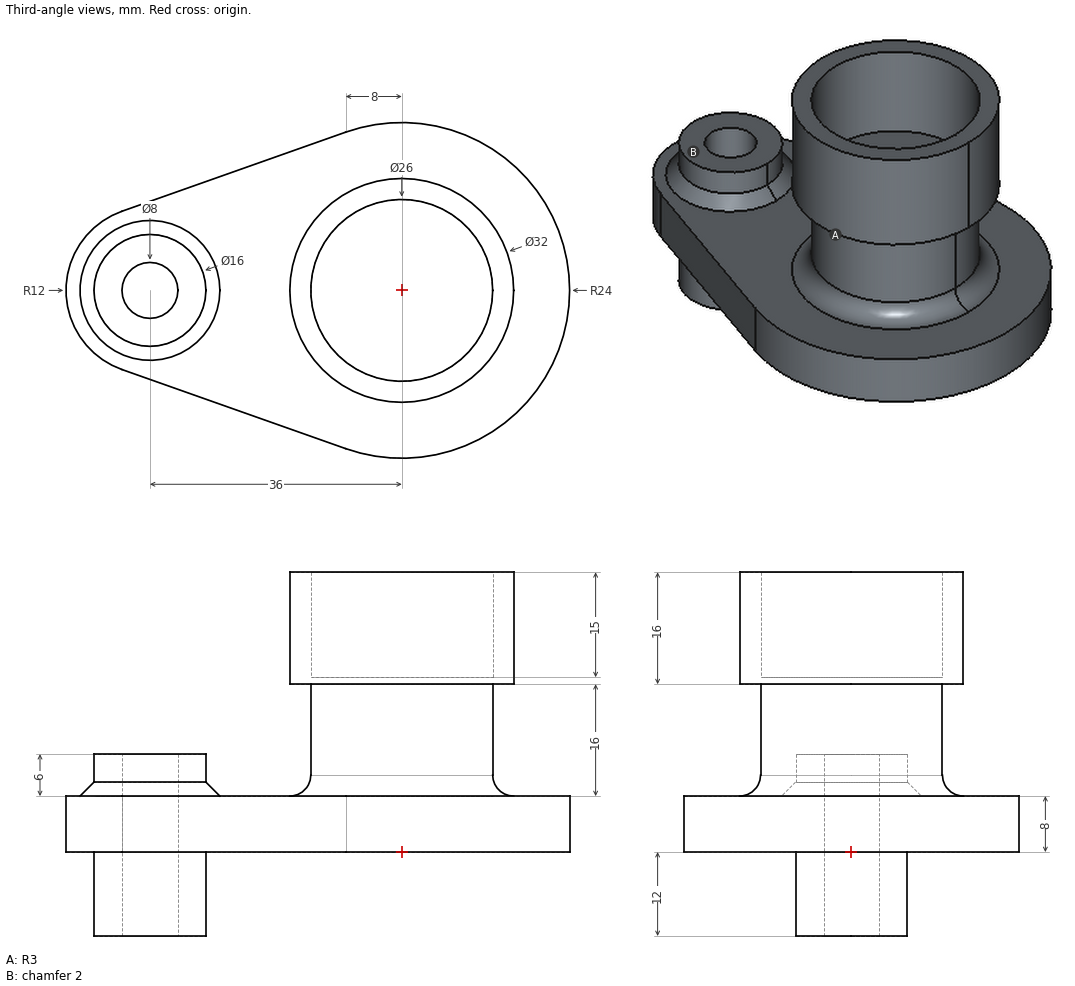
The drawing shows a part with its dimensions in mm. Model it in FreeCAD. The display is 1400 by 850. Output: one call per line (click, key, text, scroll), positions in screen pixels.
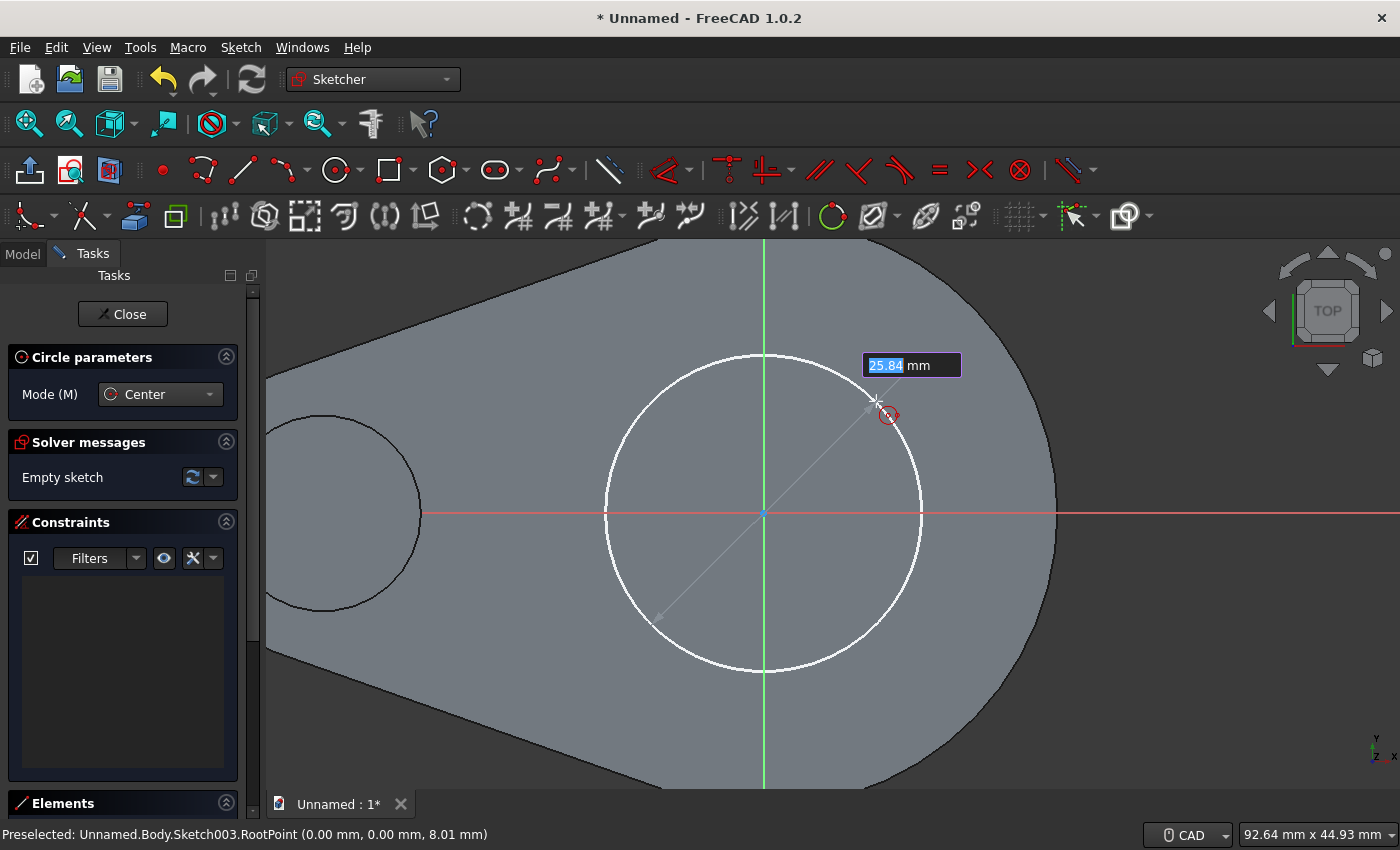
text(26)
key(Return)
key(Escape)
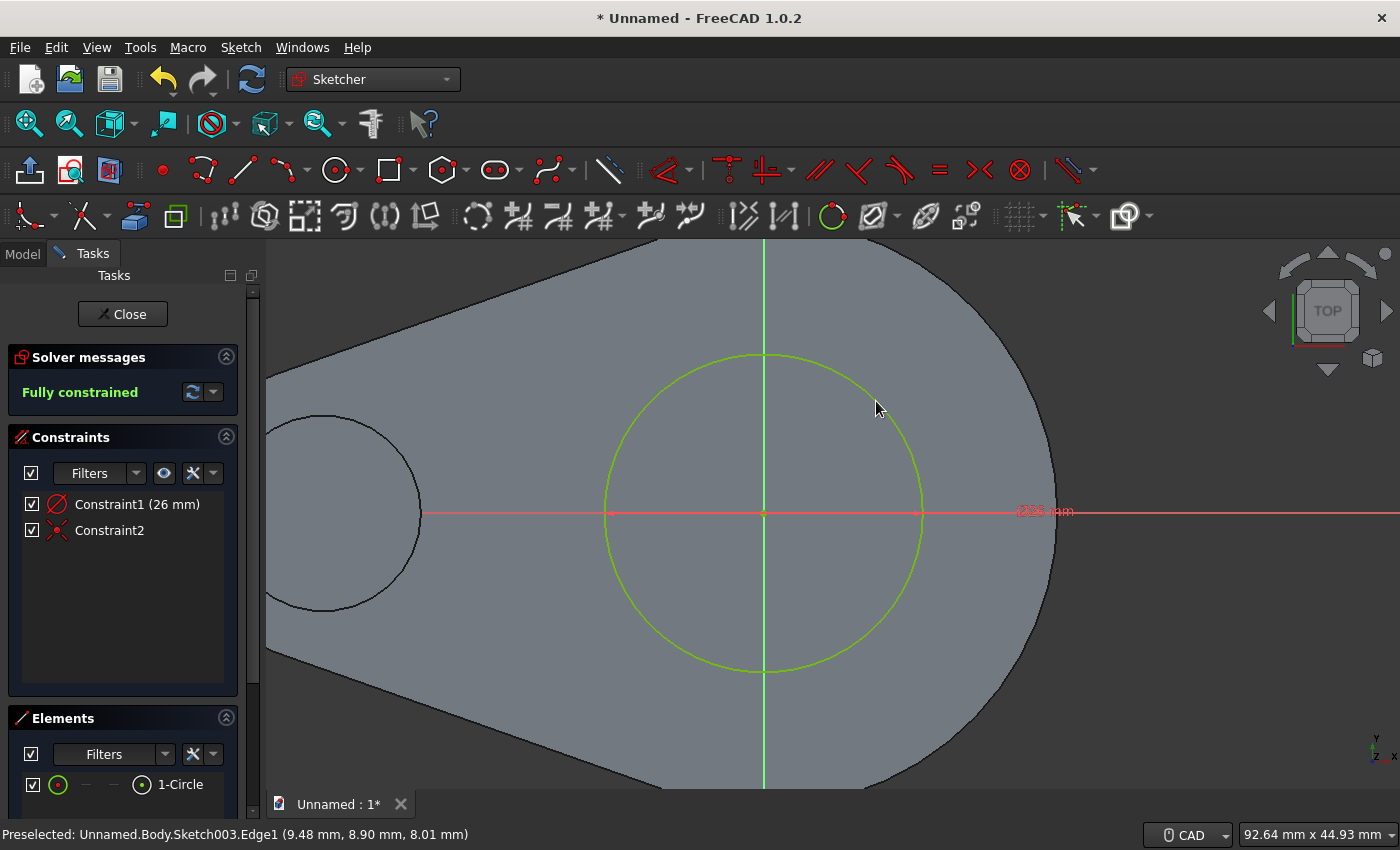
click(123, 314)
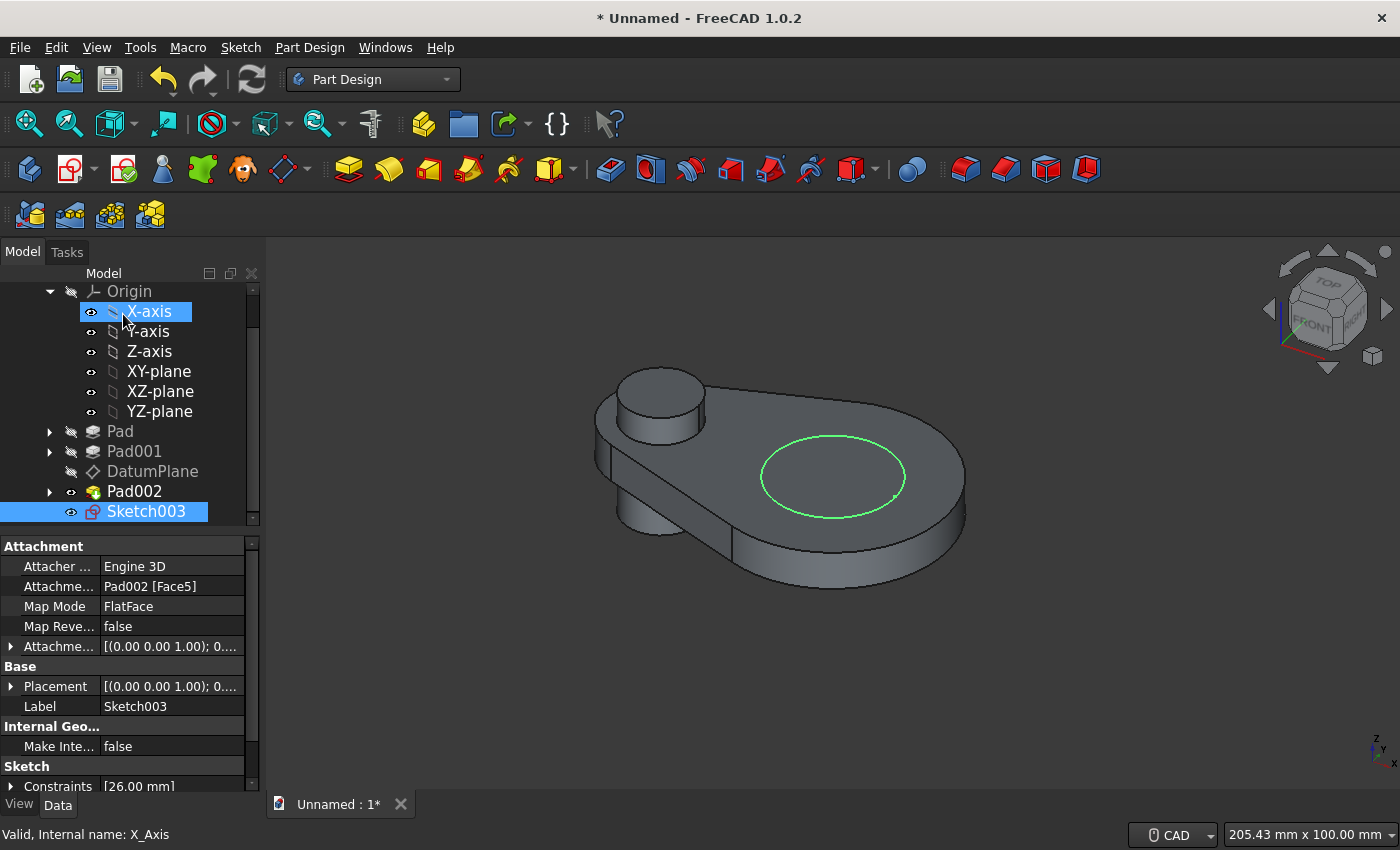
click(350, 170)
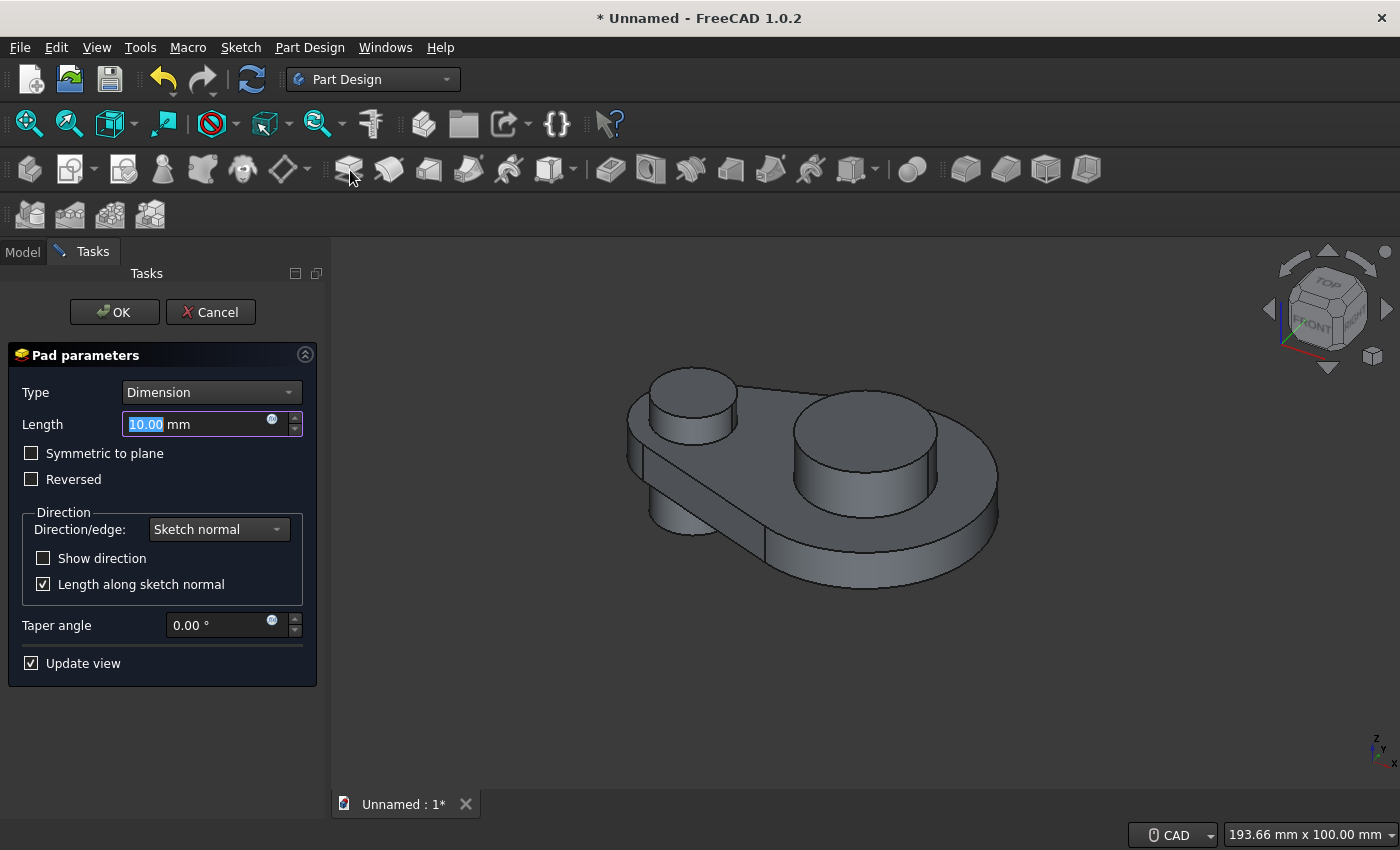
text(16)
key(Tab)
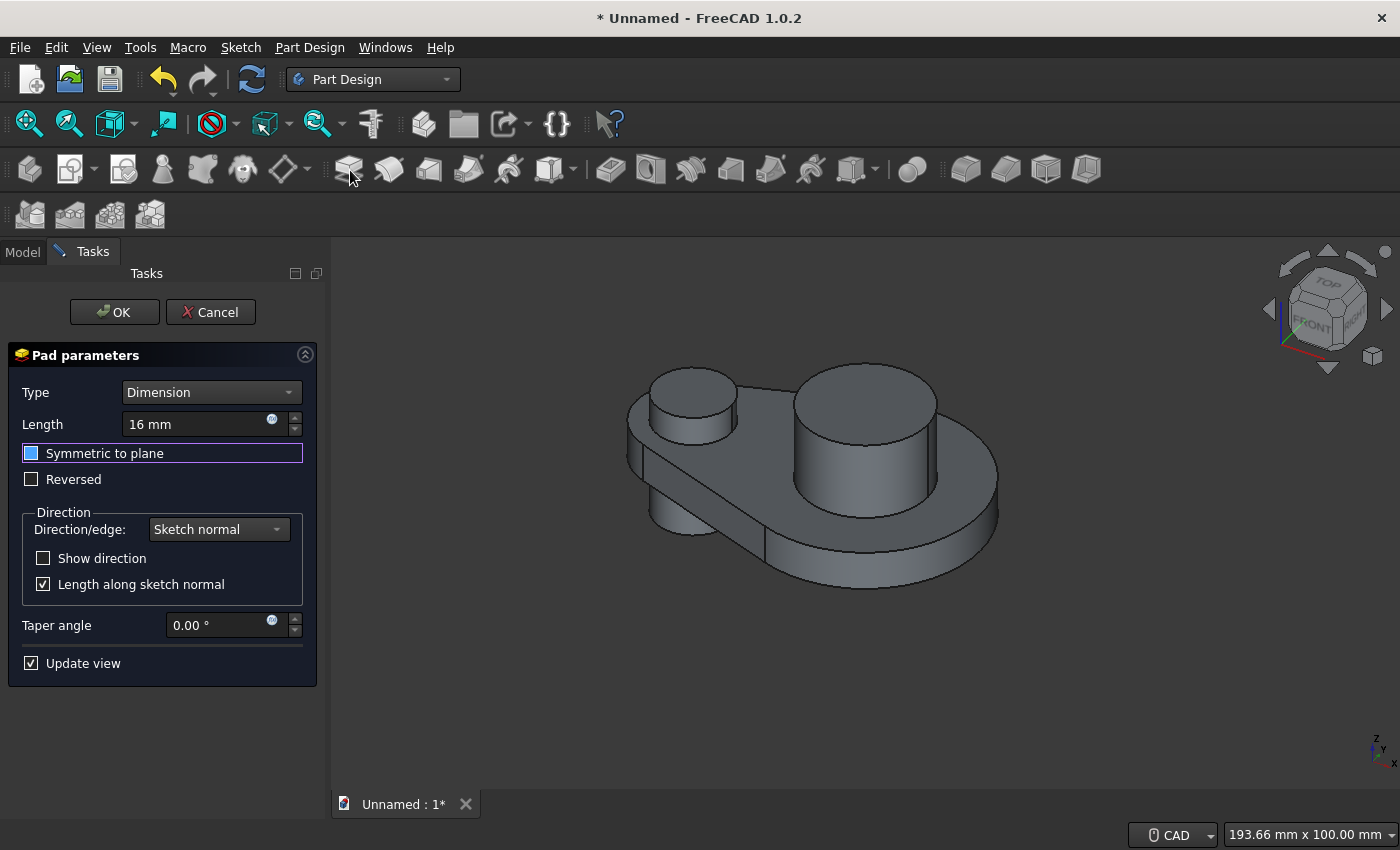
click(115, 312)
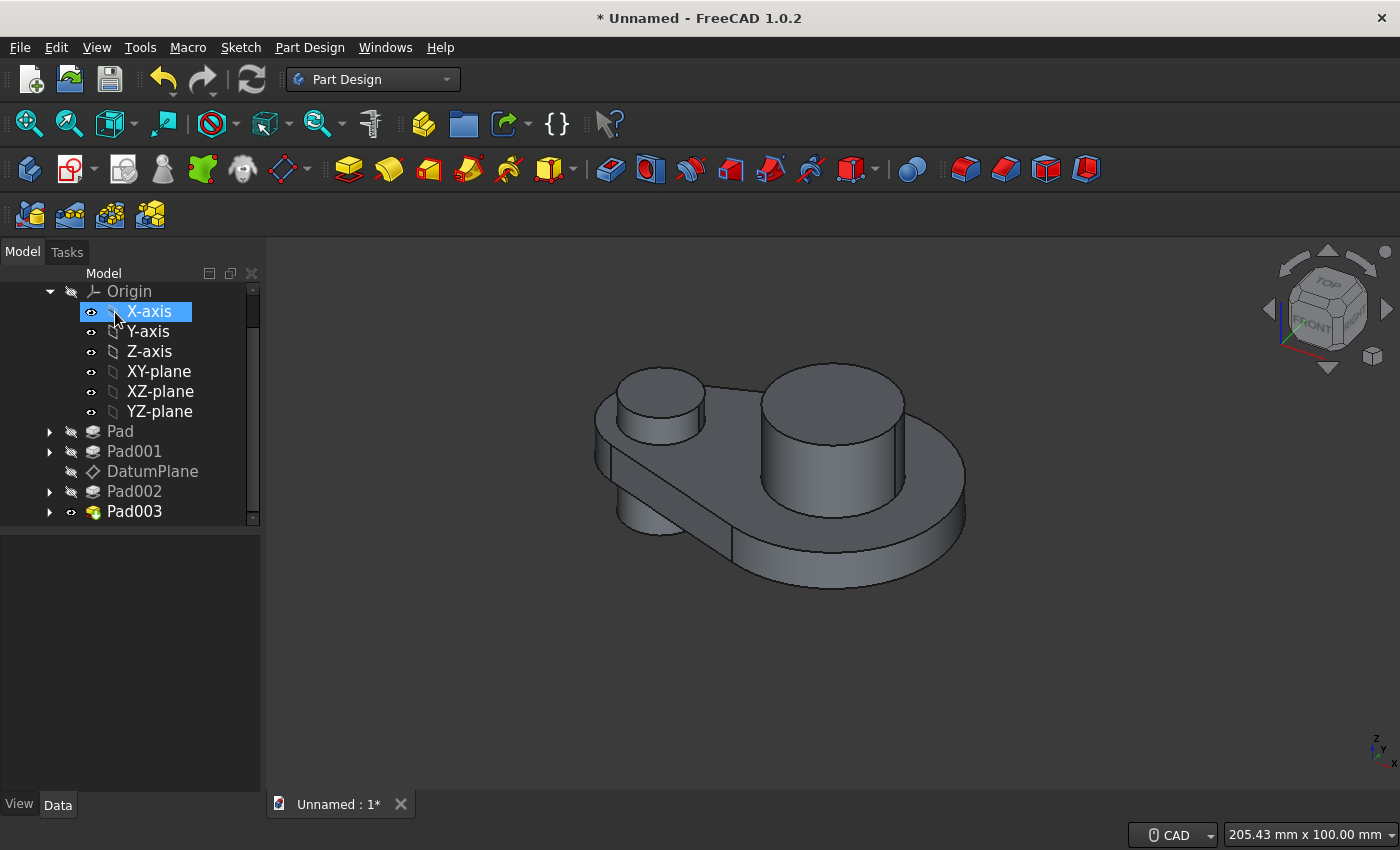
click(833, 403)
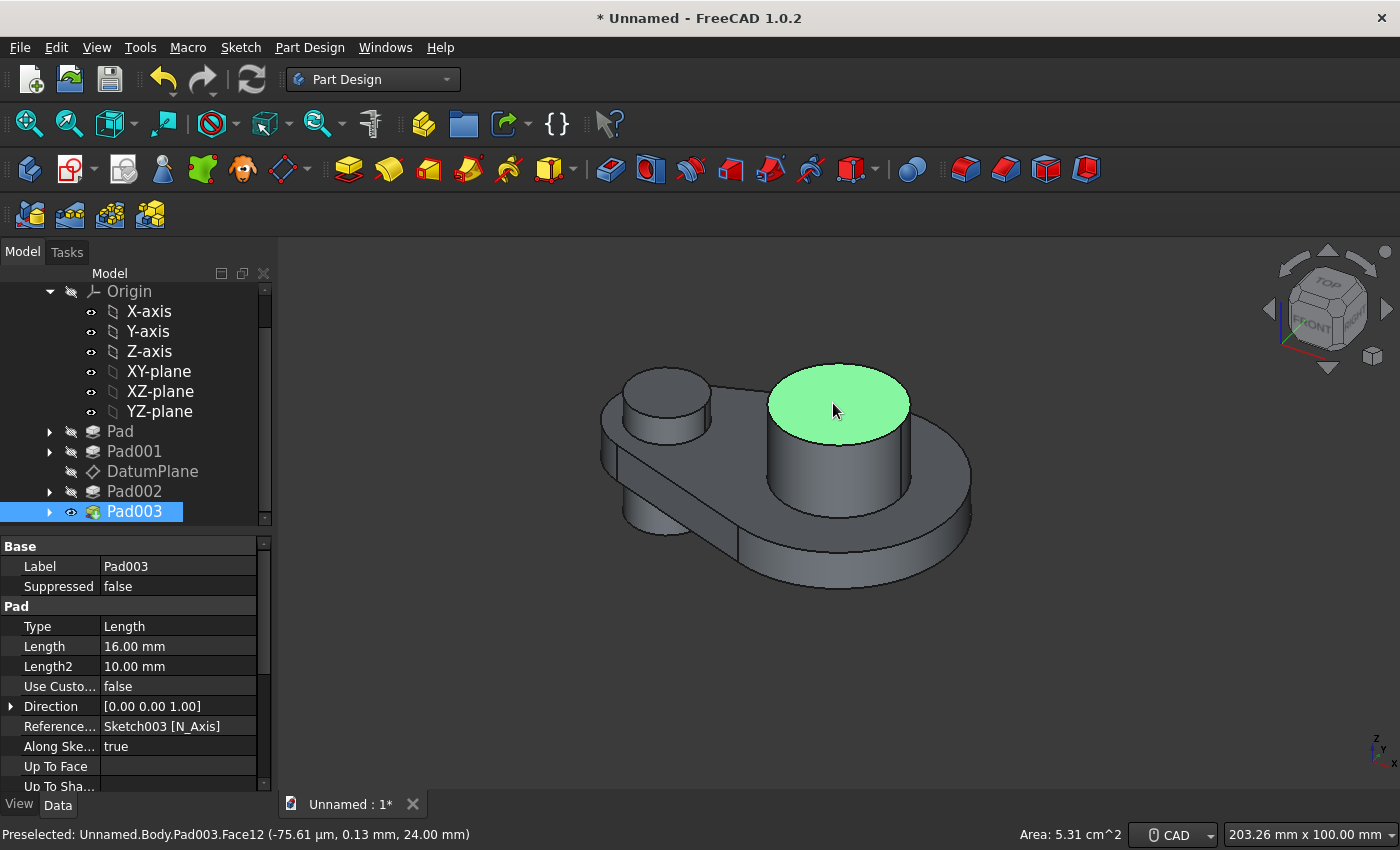
click(70, 170)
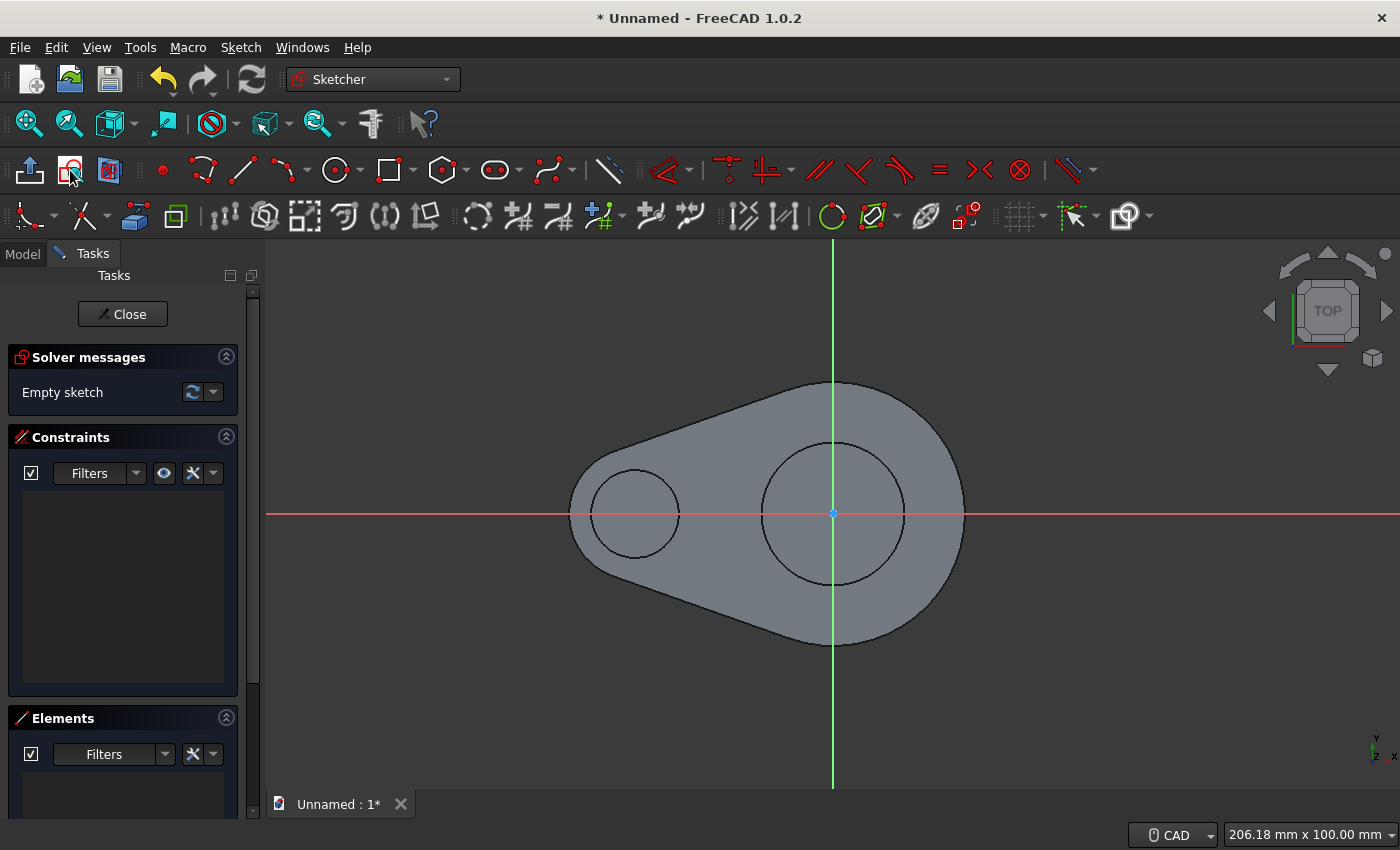
scroll(916, 514, up, 3)